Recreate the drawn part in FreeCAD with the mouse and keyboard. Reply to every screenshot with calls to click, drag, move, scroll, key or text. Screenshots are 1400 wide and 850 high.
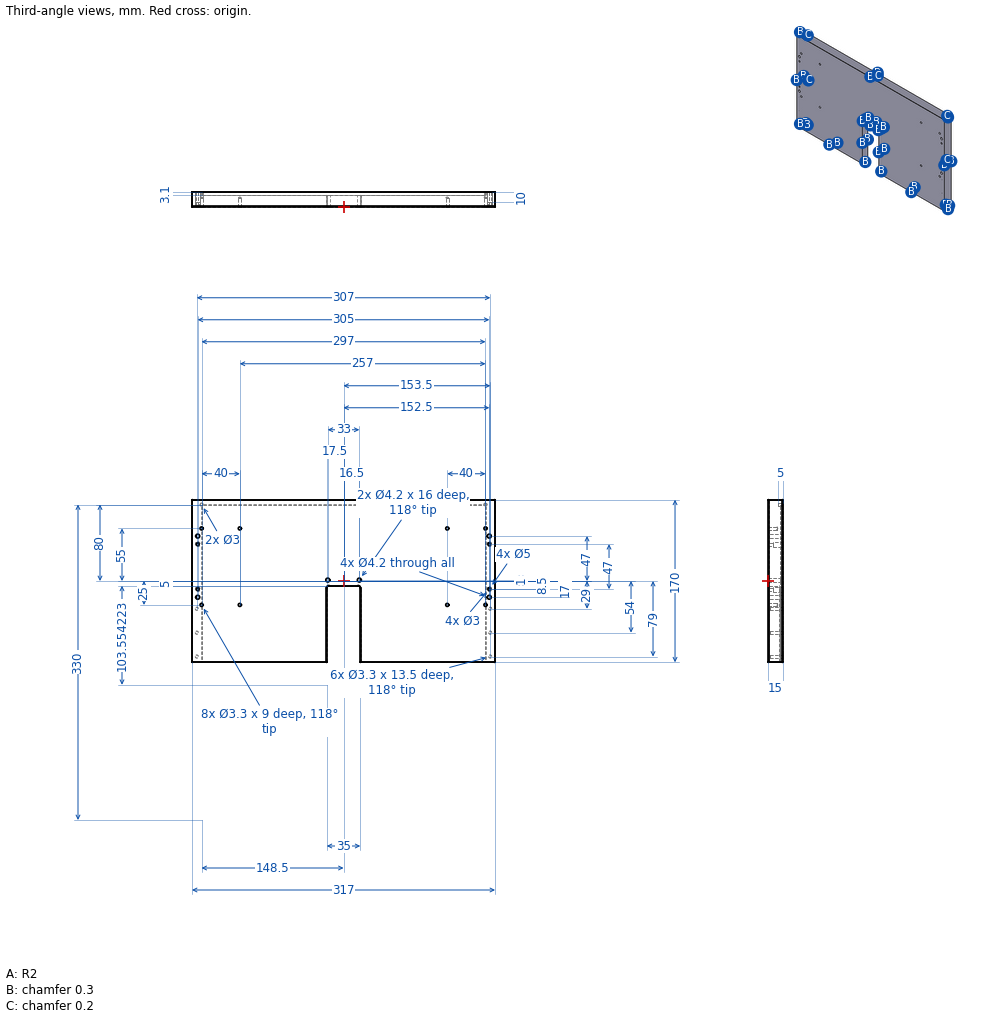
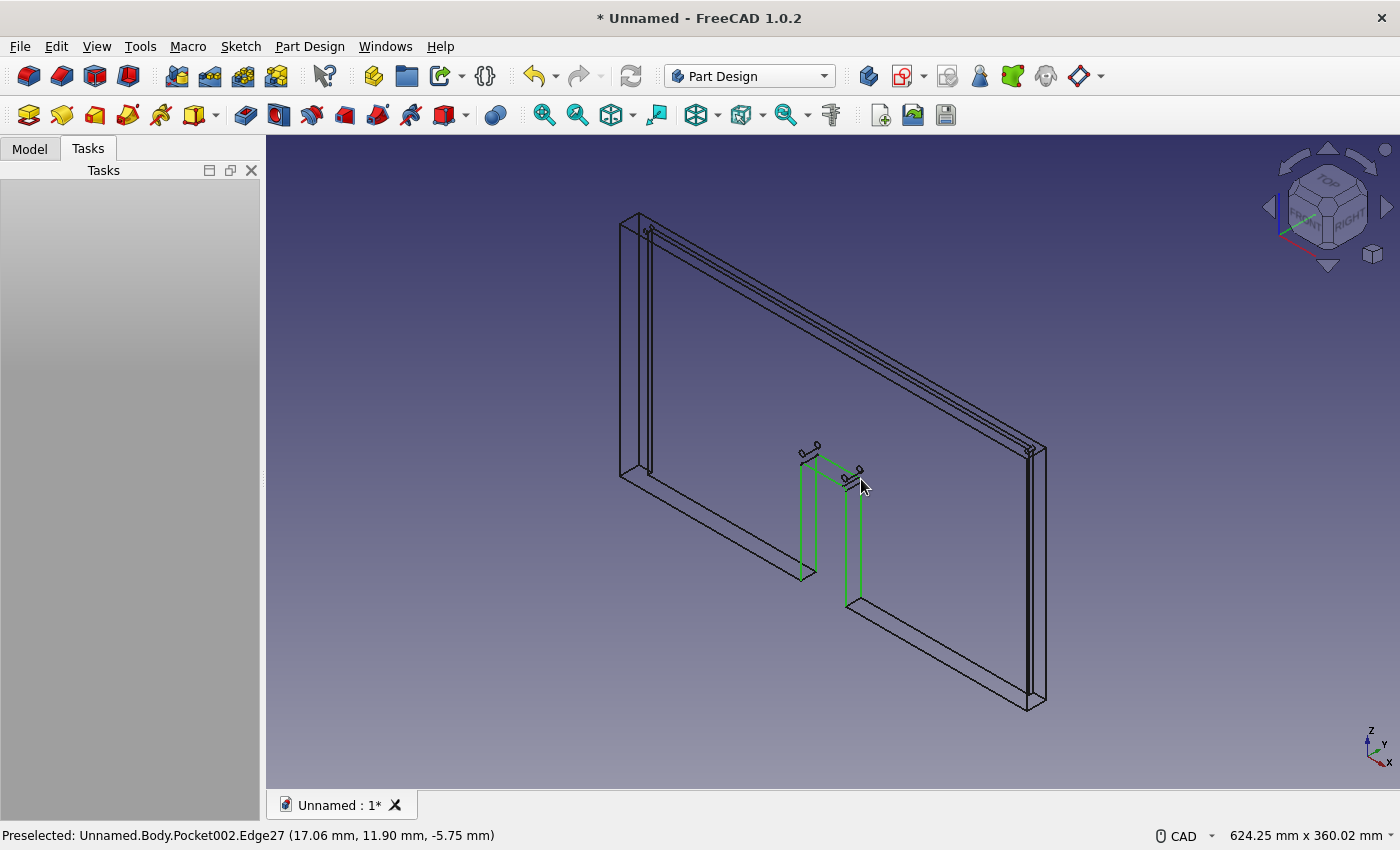
scroll(802, 462, up, 10)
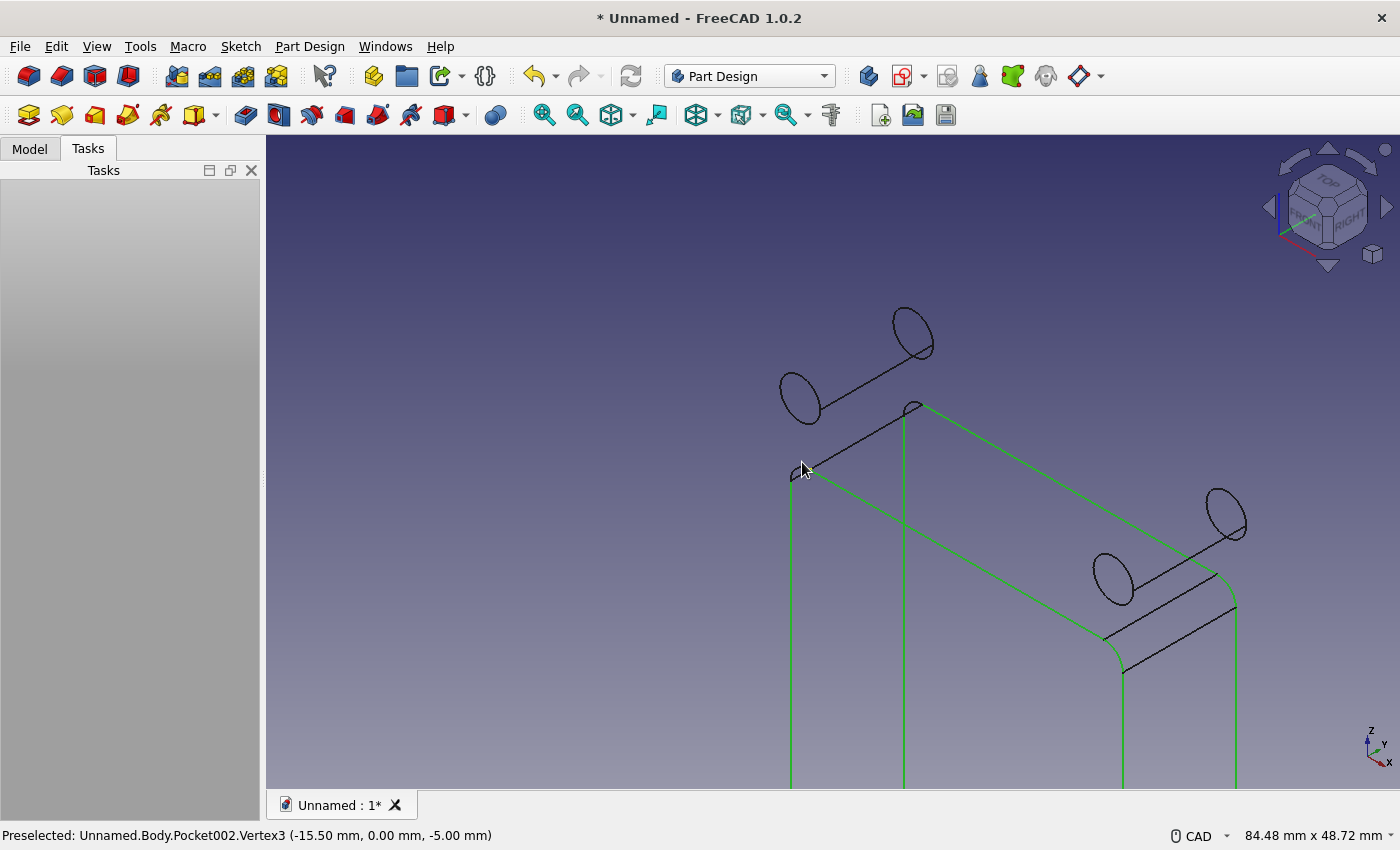
click(796, 467, ctrl)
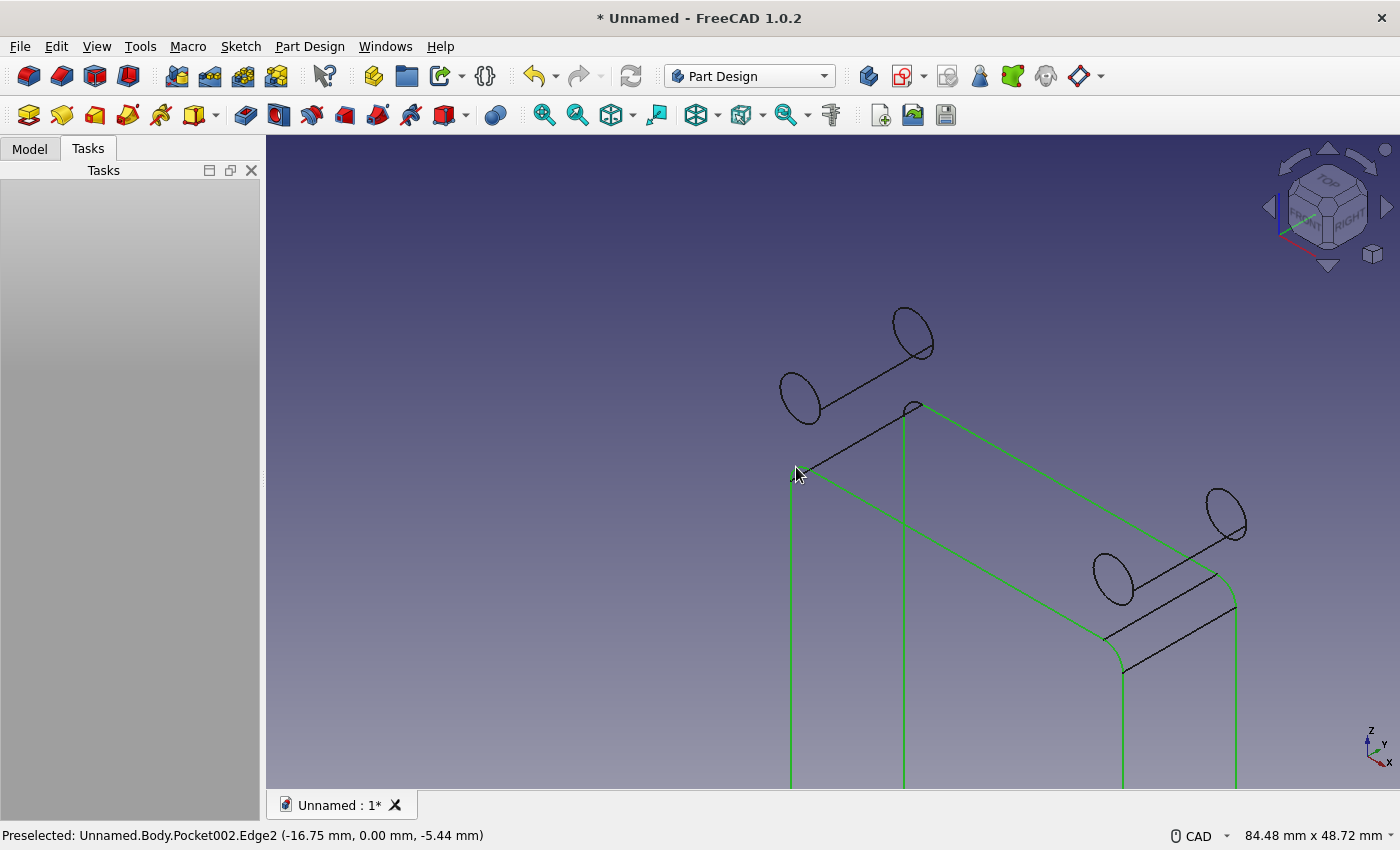
click(909, 402, ctrl)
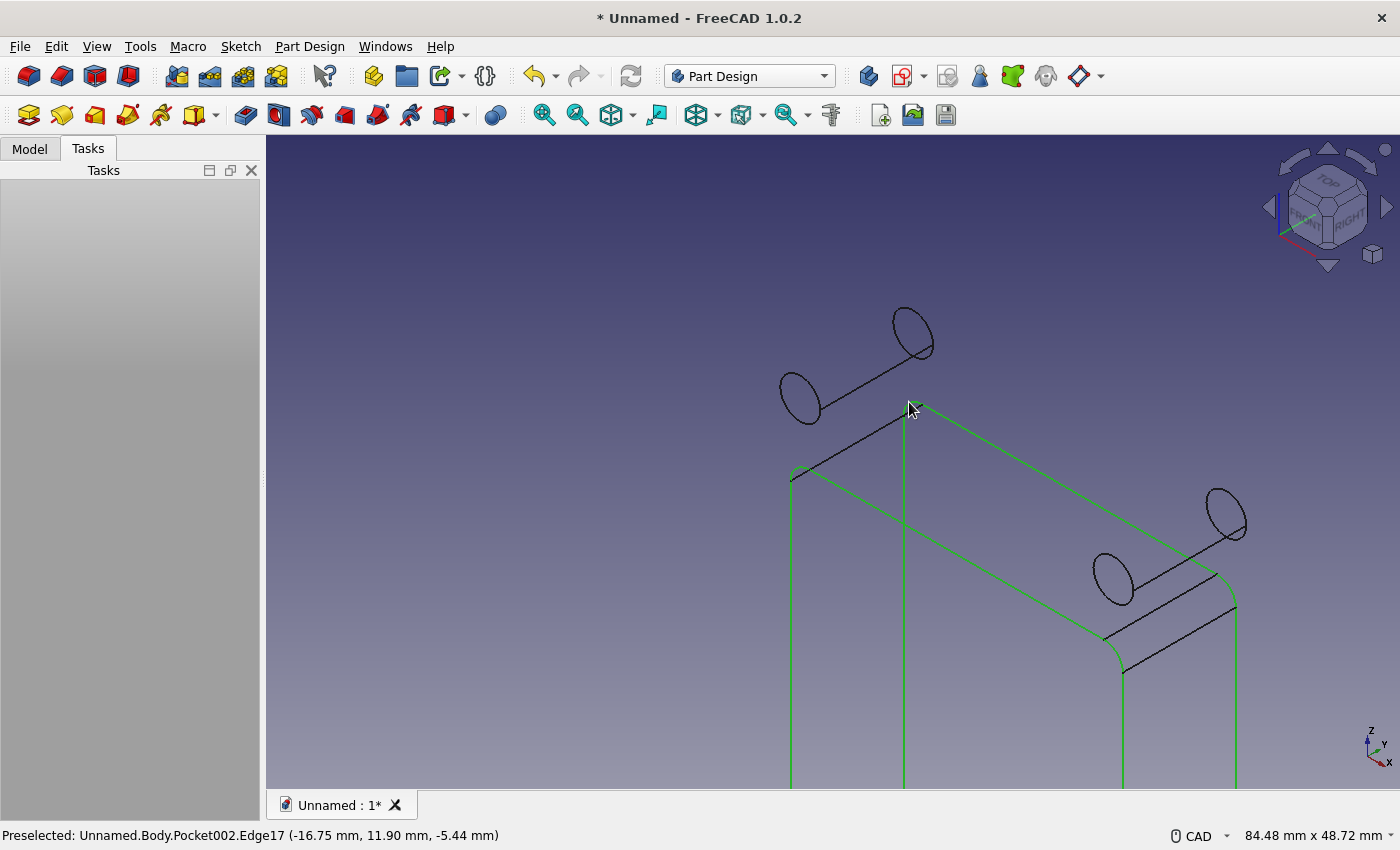
key(v)
key(1)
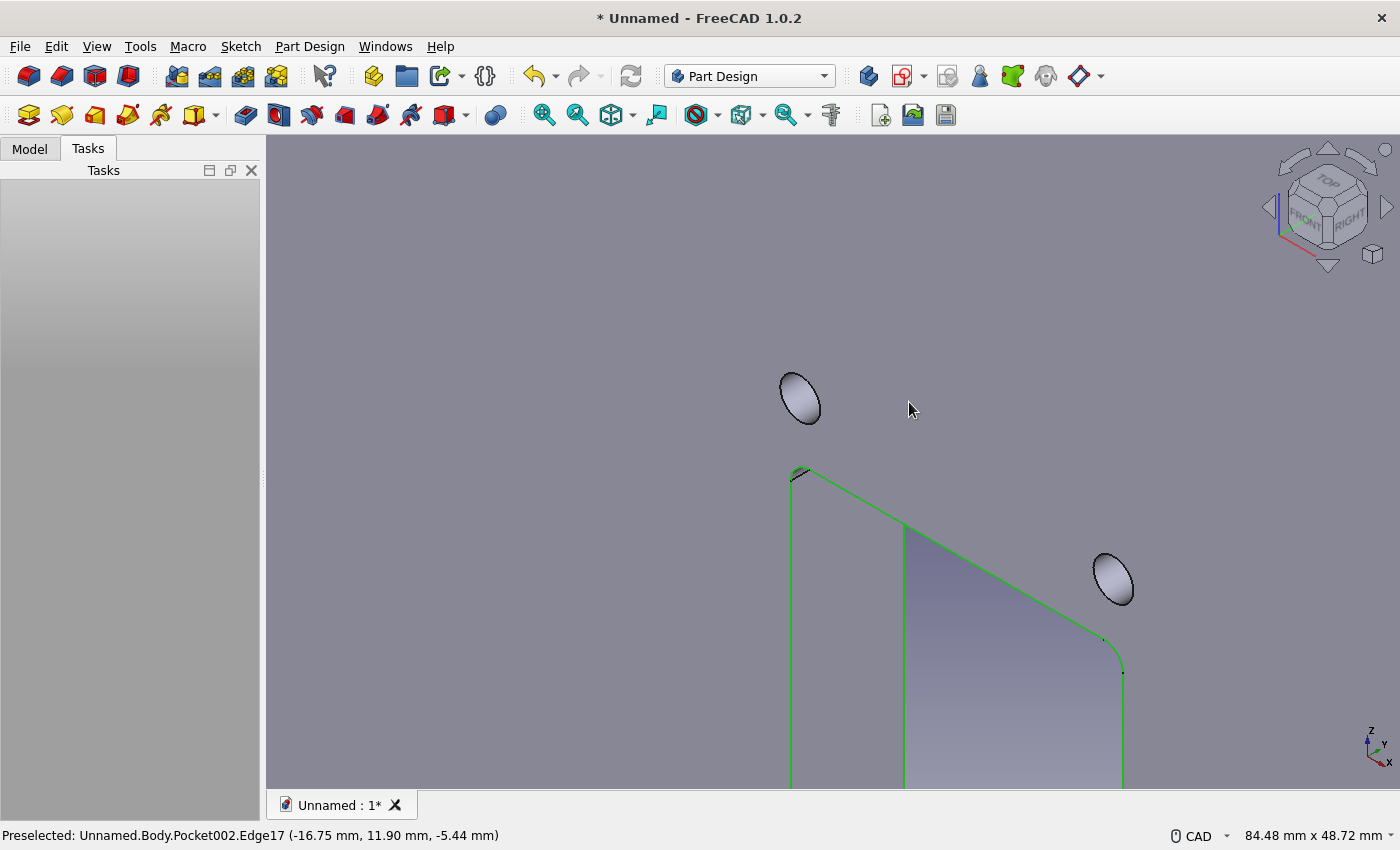
click(62, 76)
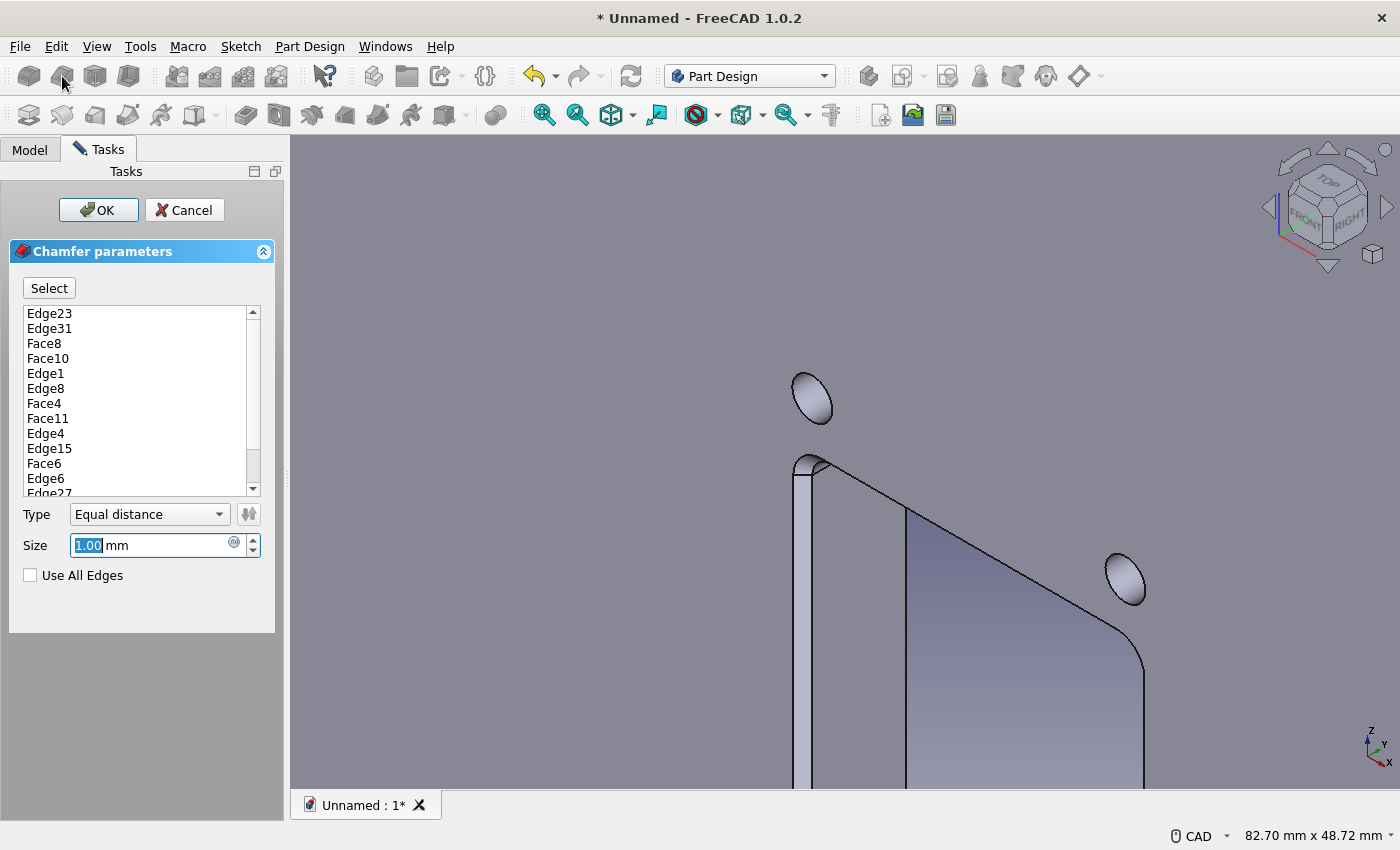
text(0.3)
key(Tab)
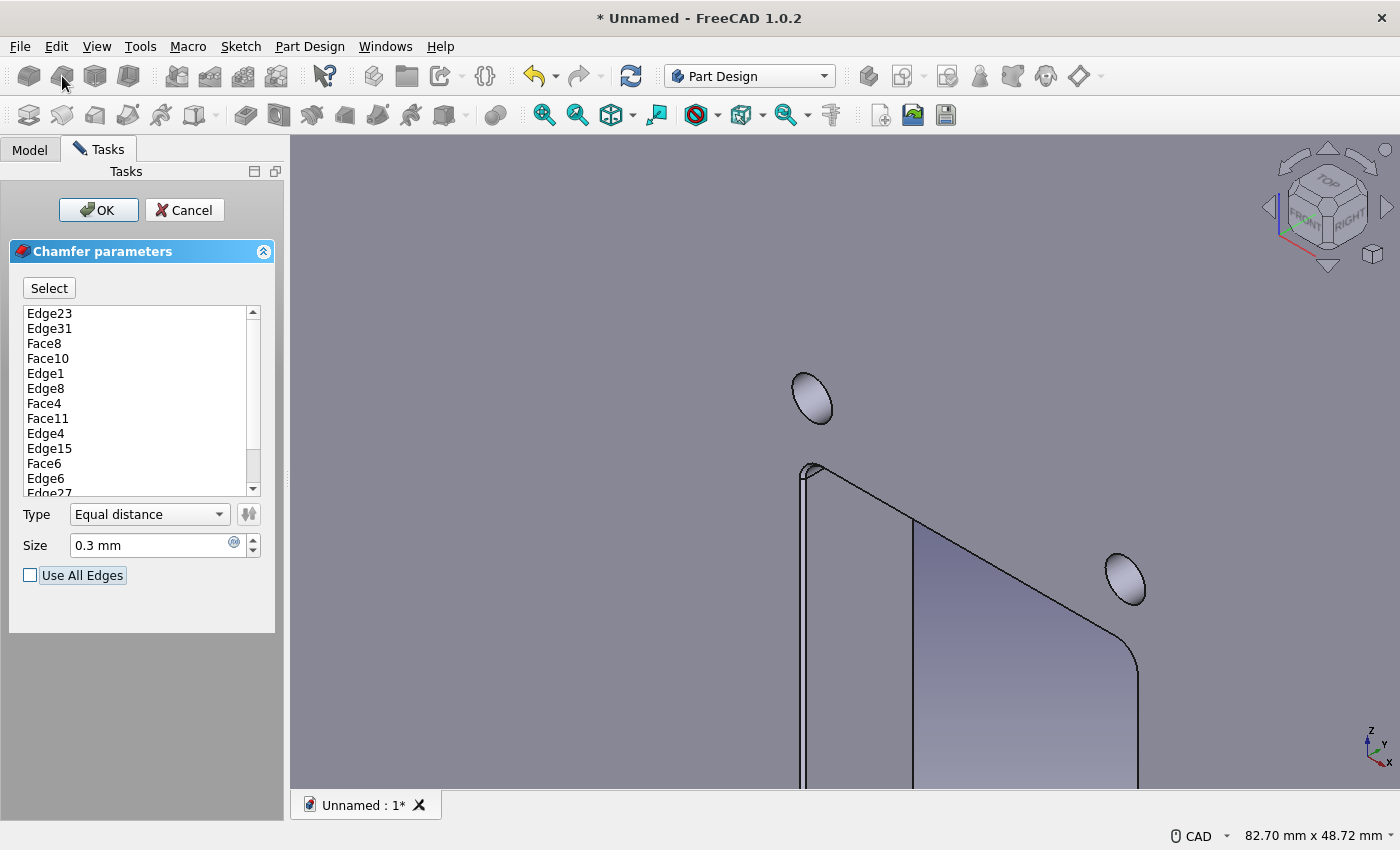
click(99, 210)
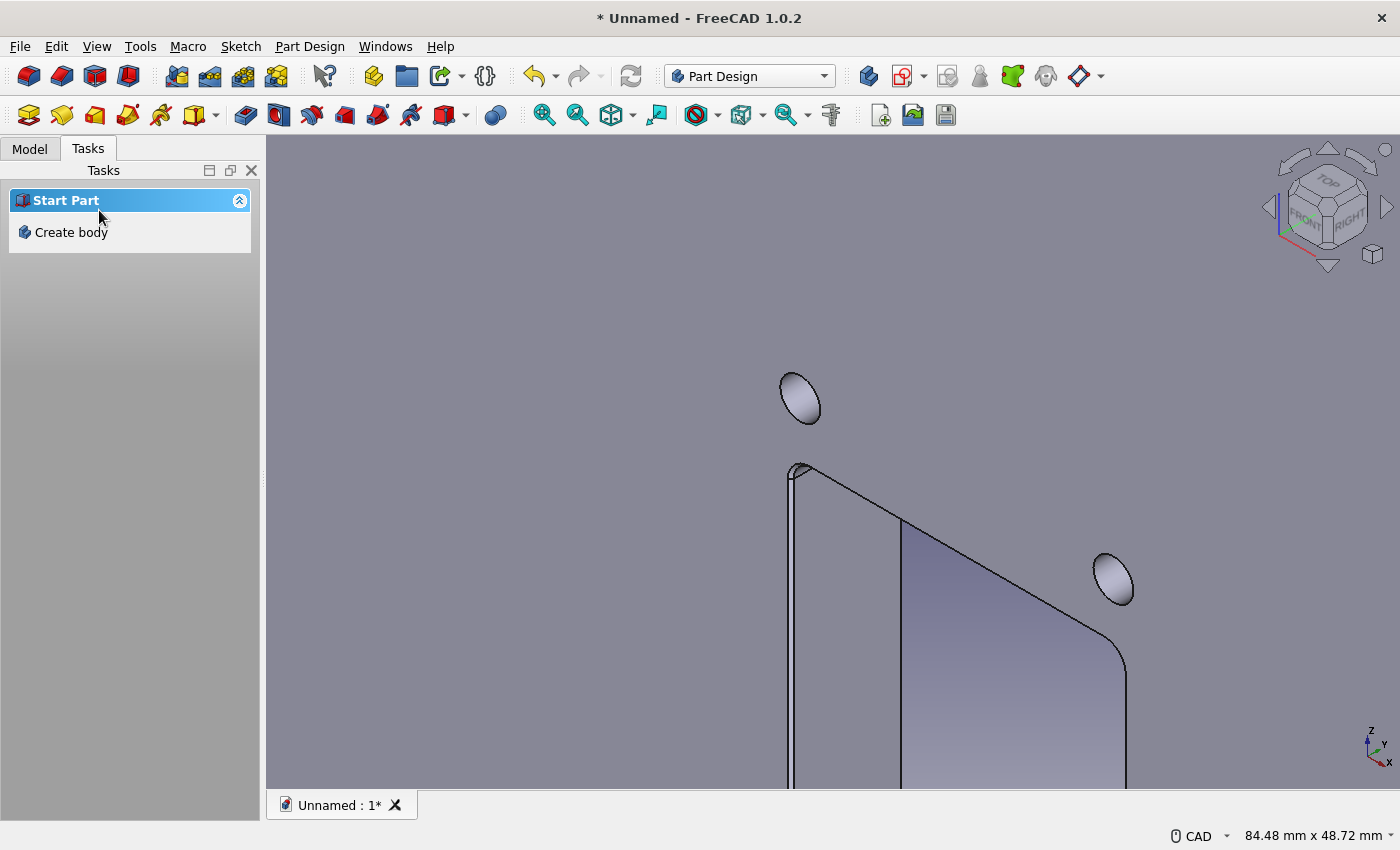
key(v)
key(f)